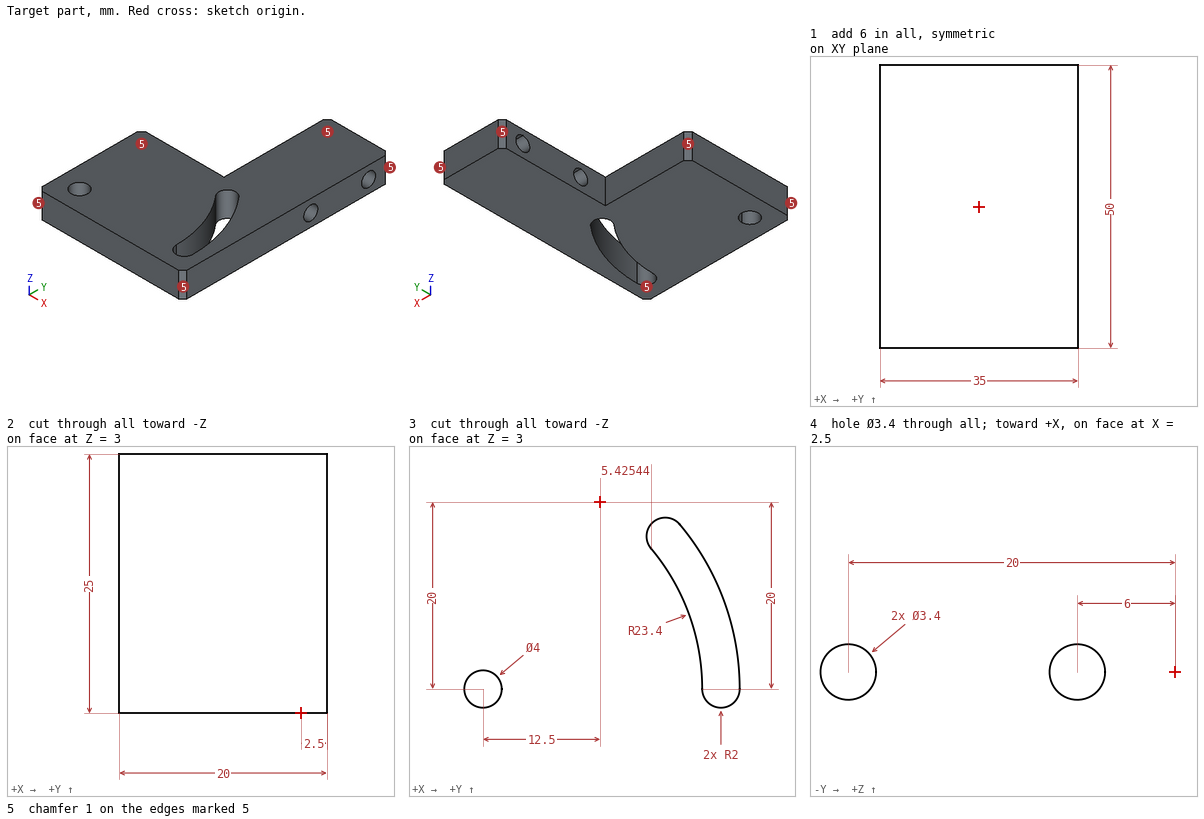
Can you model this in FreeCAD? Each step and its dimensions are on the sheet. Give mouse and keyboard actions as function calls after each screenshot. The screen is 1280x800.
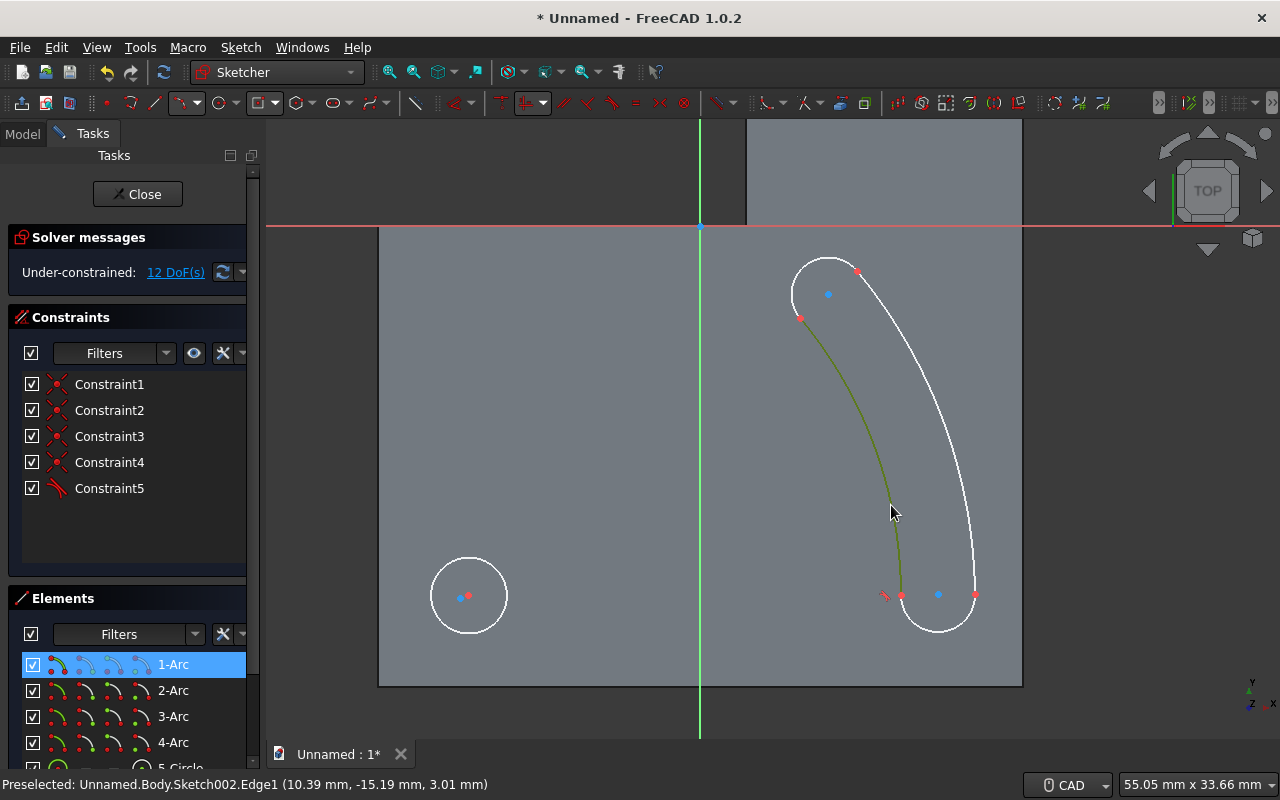
click(826, 258)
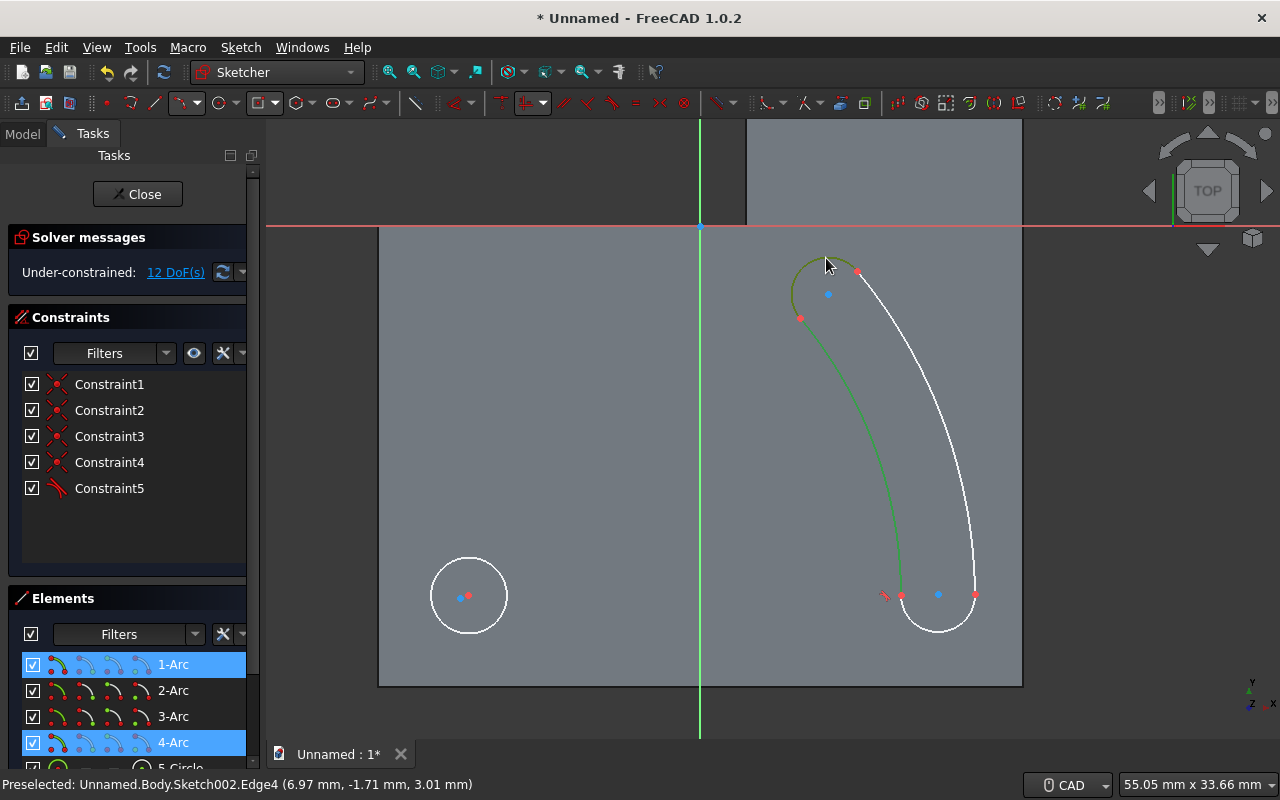
key(t)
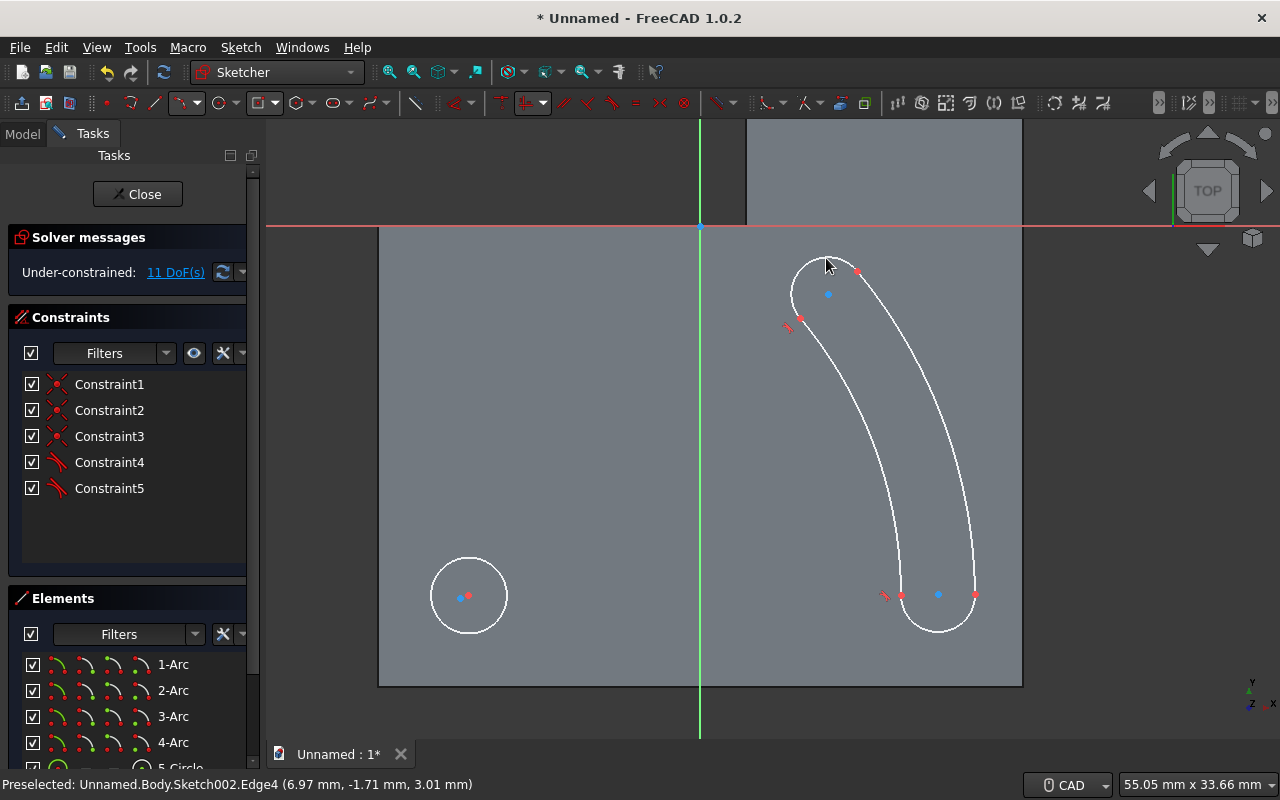
click(916, 625)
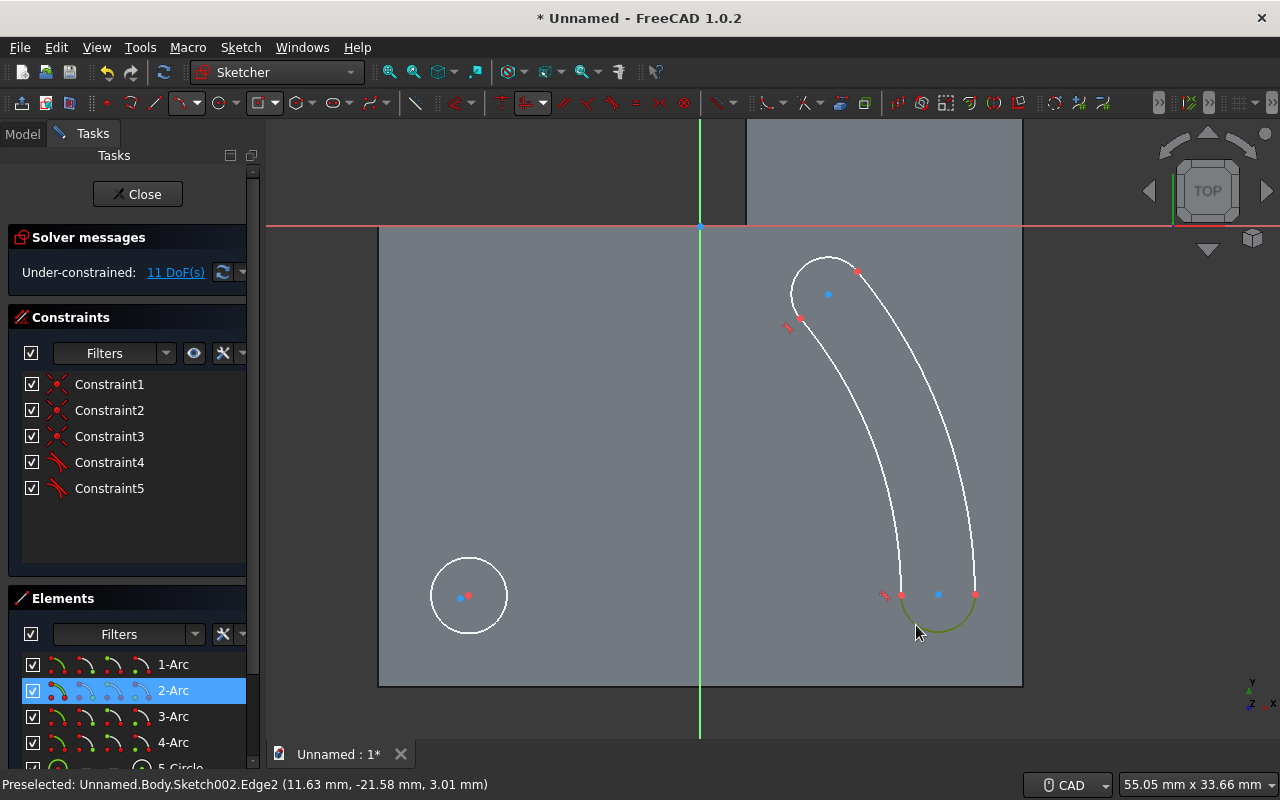
click(963, 490)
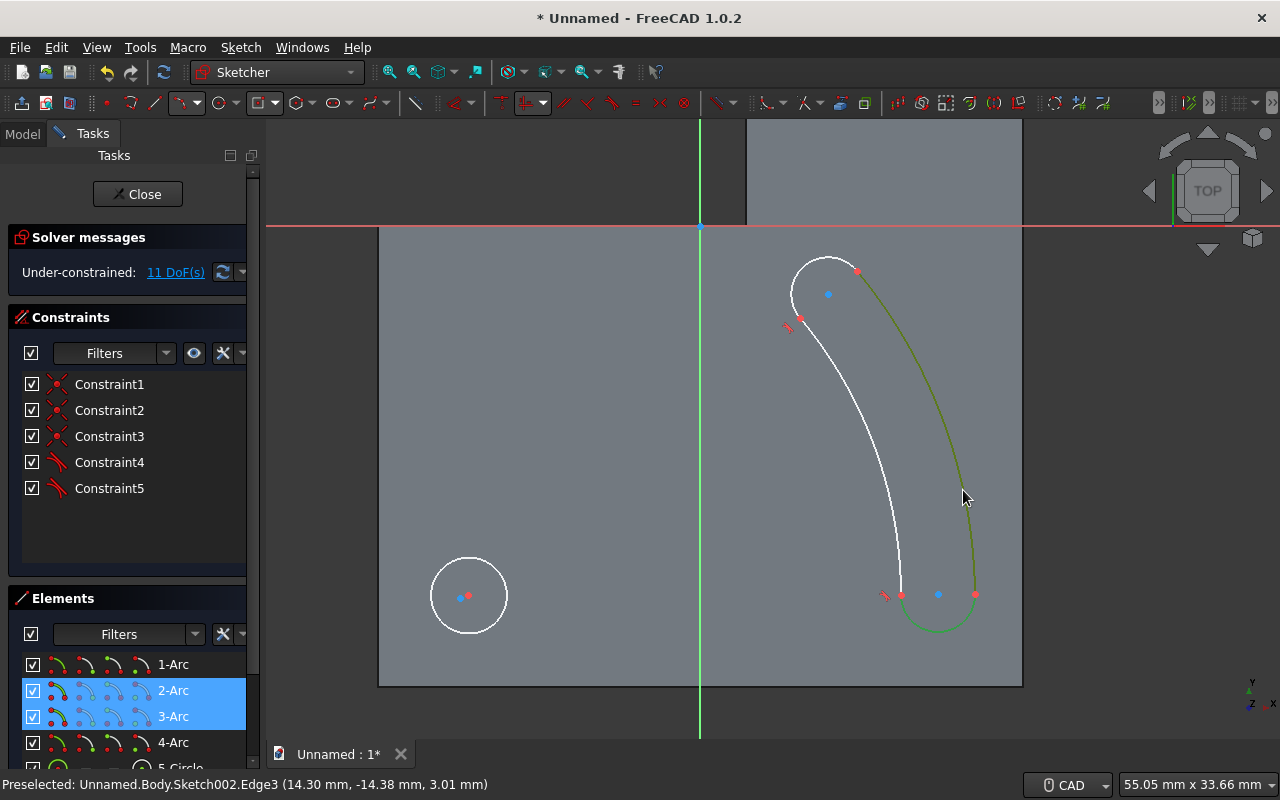
click(612, 104)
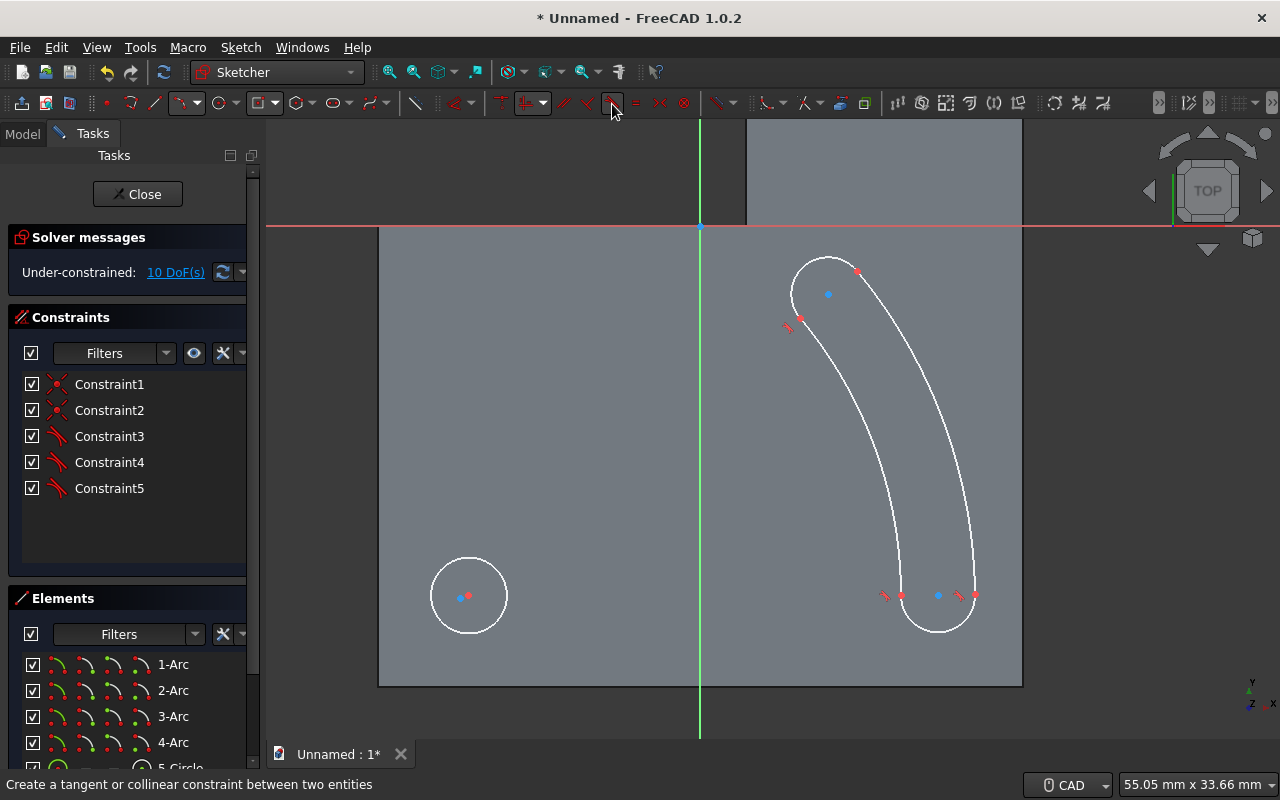
click(963, 490)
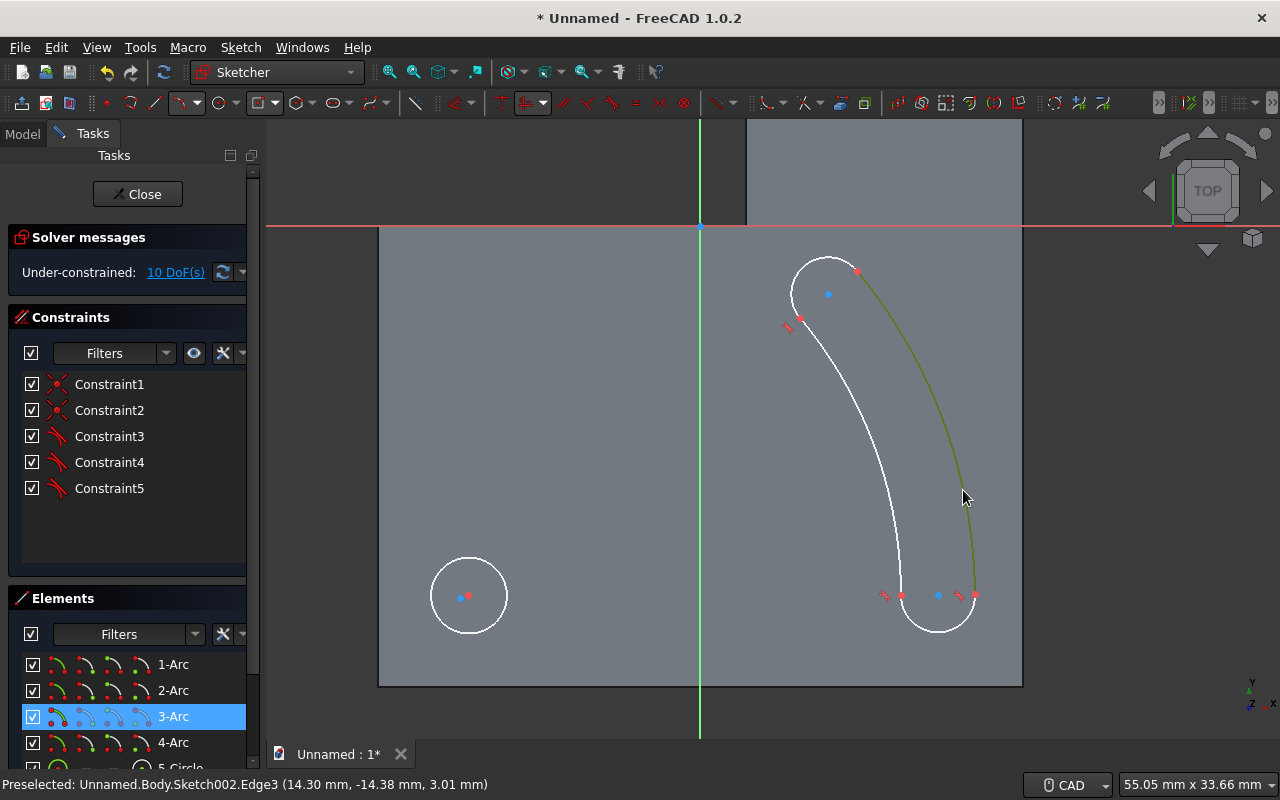
click(826, 257)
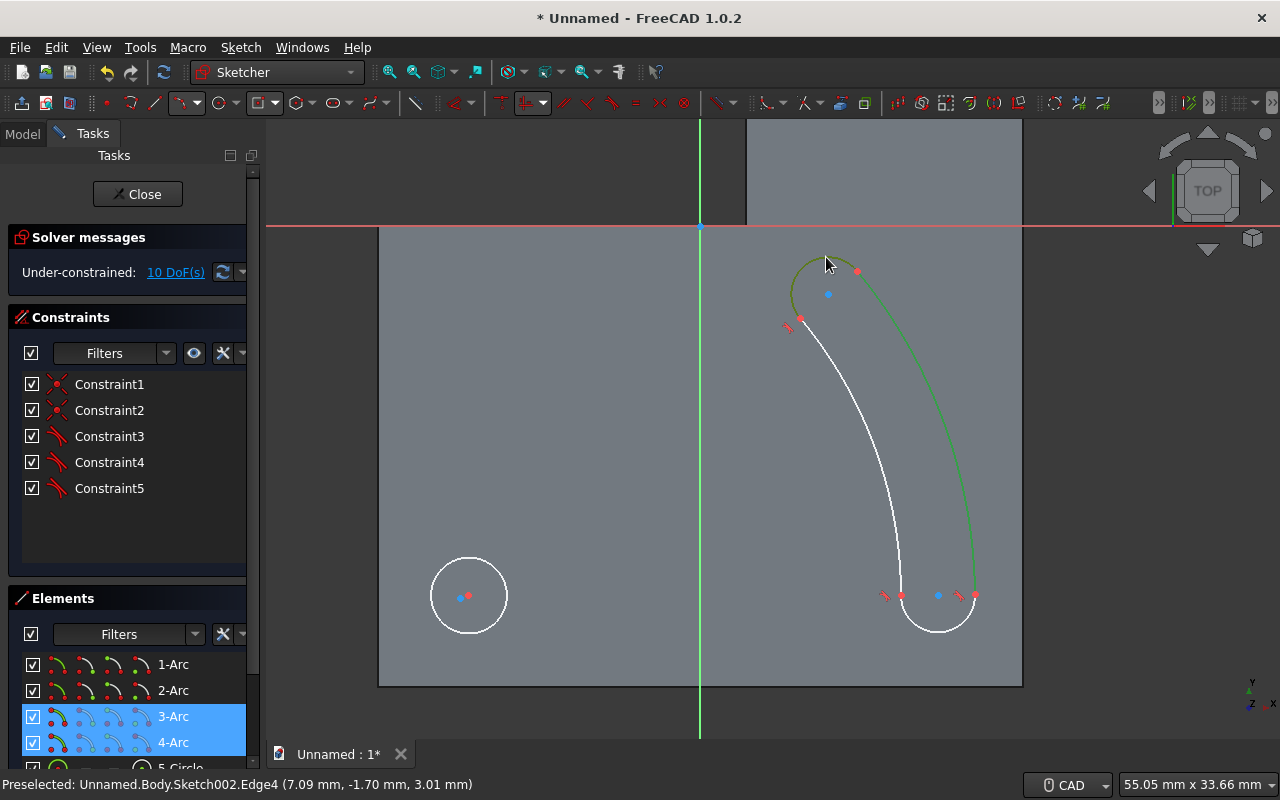
click(612, 104)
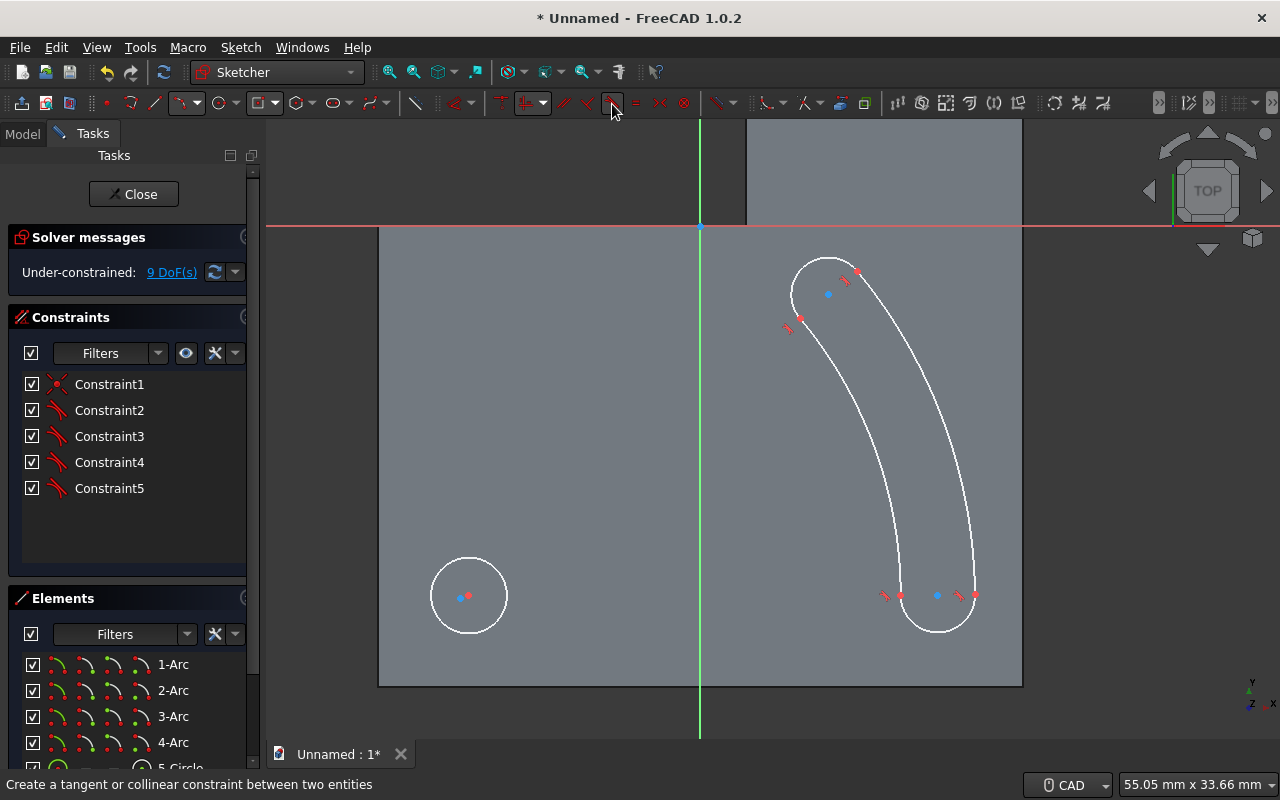
click(496, 569)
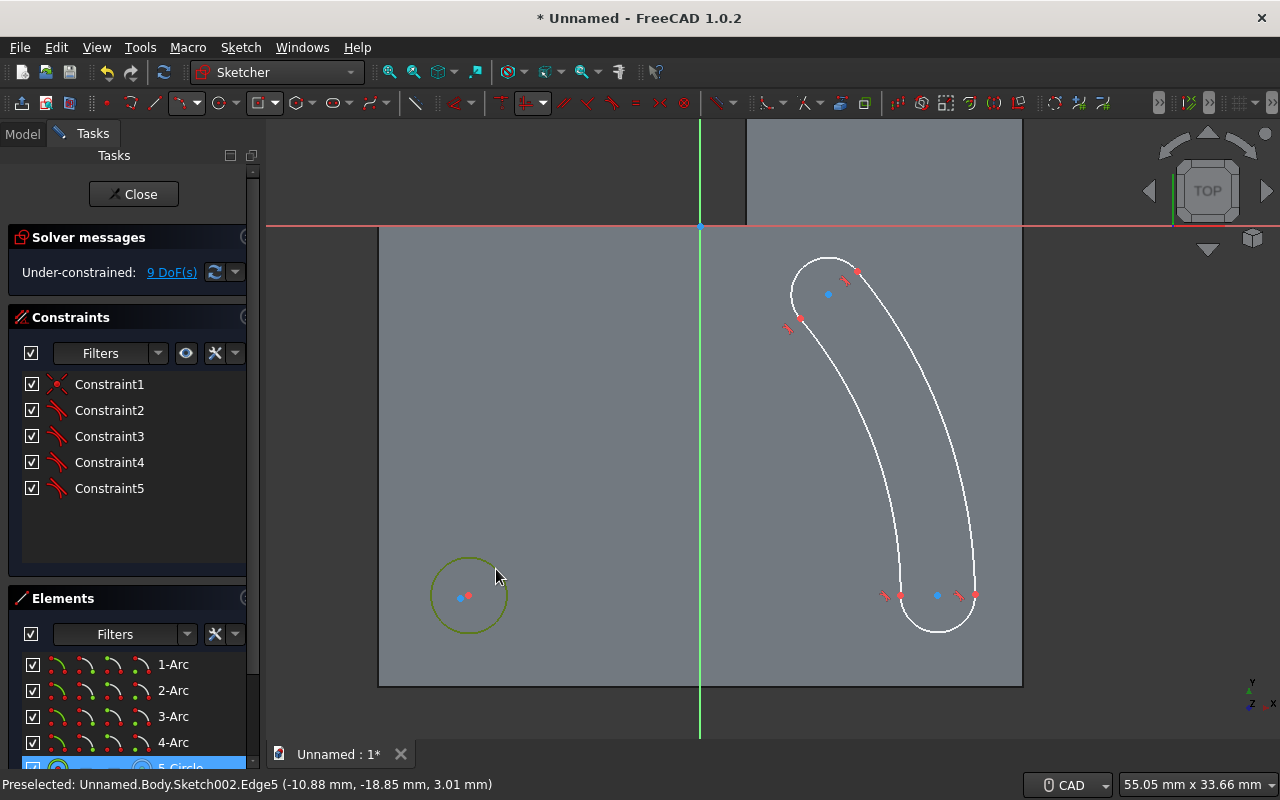
click(963, 490)